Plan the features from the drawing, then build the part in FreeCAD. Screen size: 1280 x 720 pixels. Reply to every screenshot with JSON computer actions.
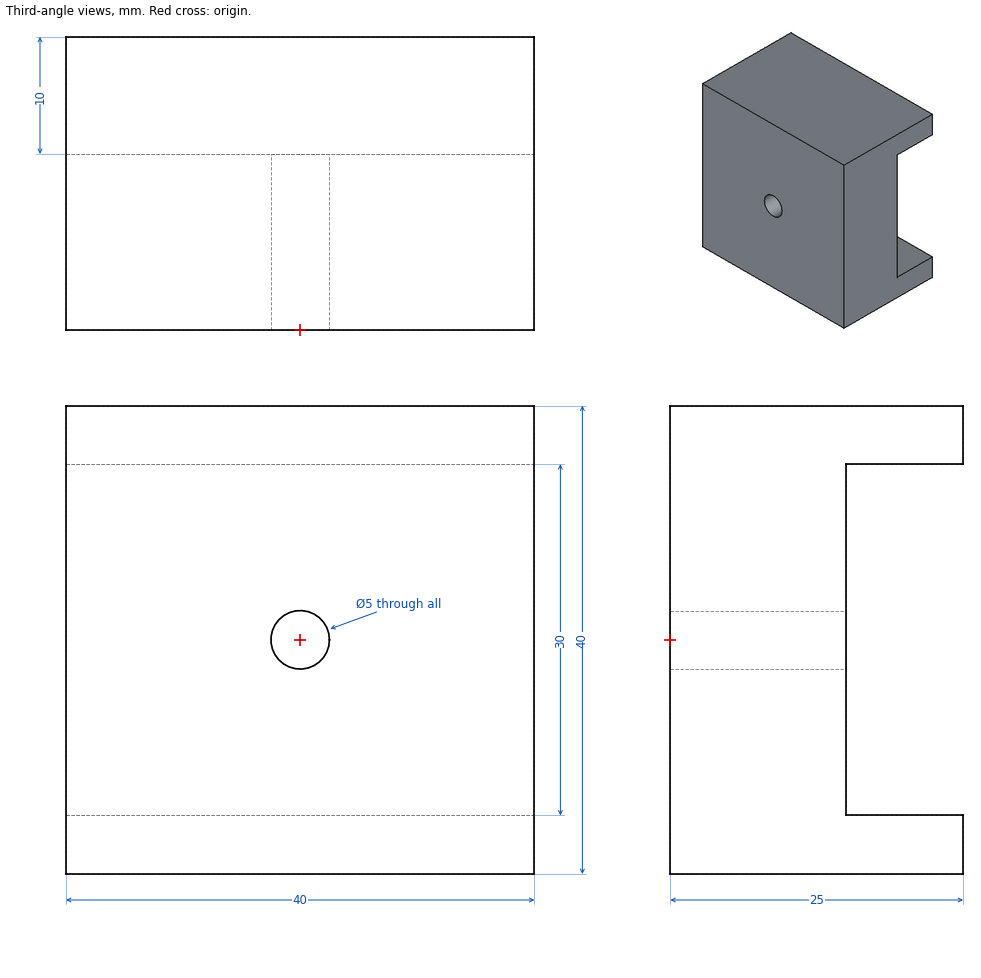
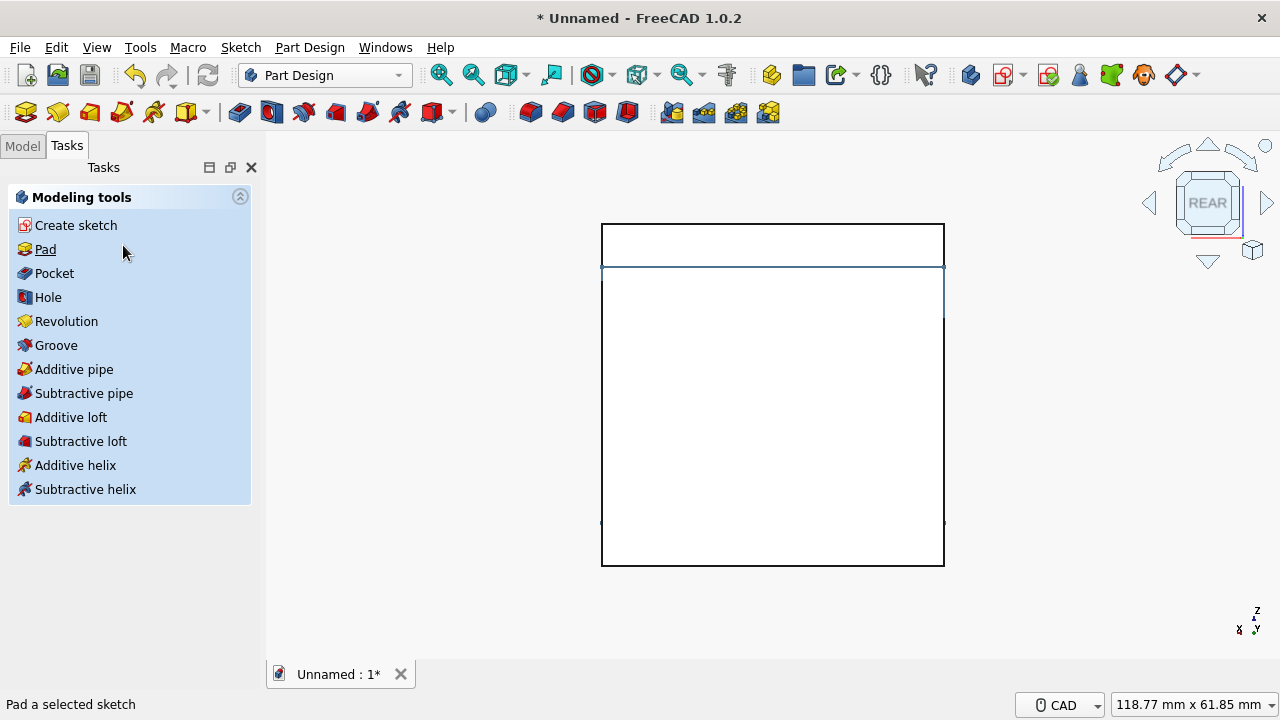
{"action": "left_click", "coordinate": [240, 112]}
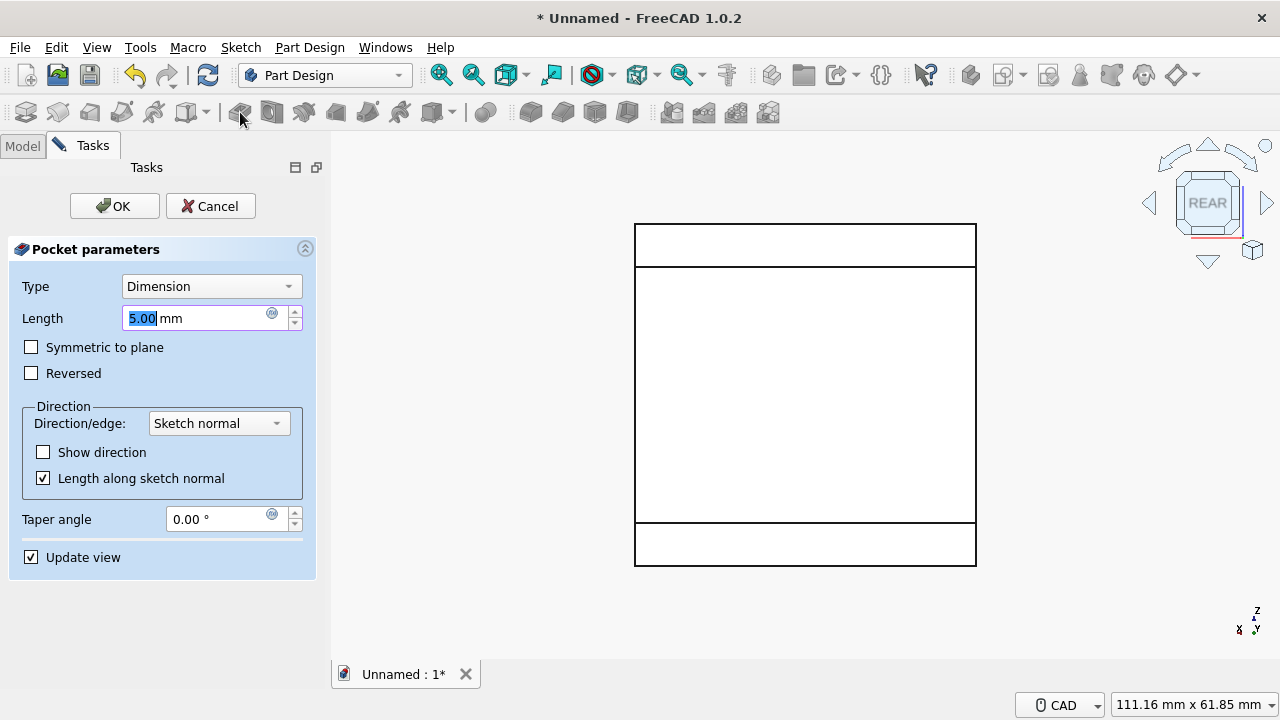
{"action": "type", "text": "10"}
{"action": "key", "text": "Tab"}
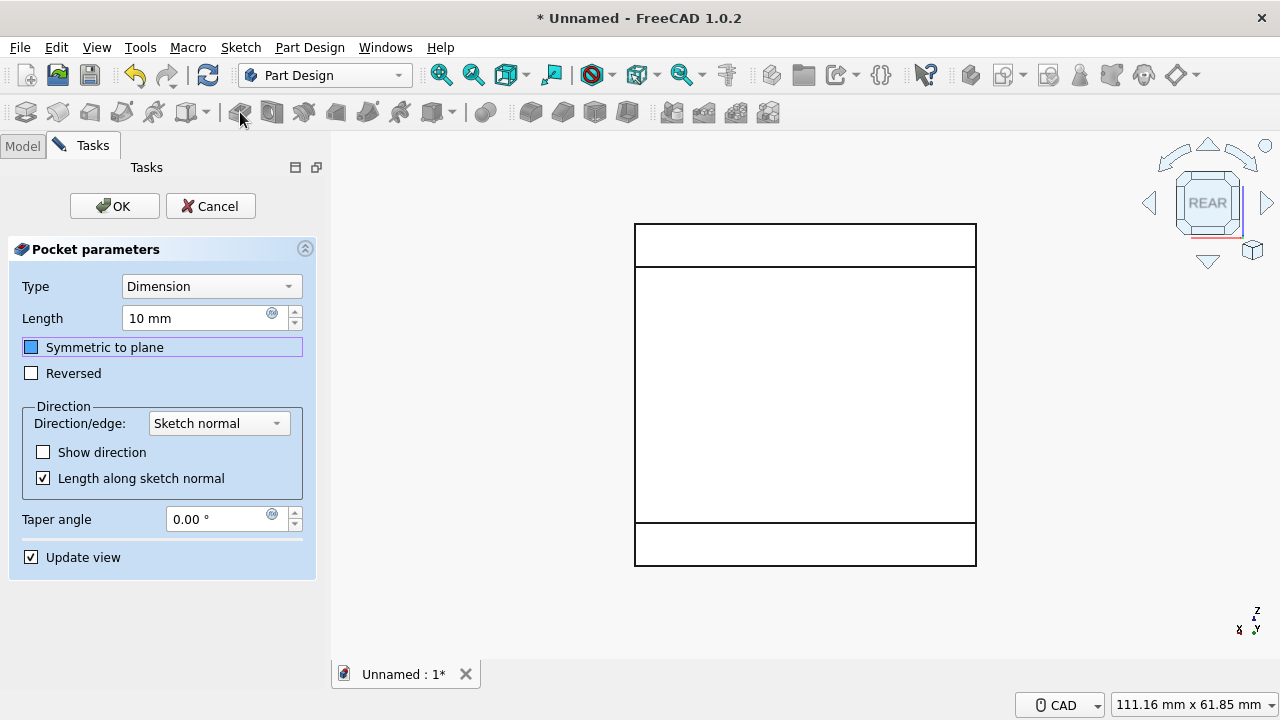
{"action": "left_click", "coordinate": [115, 206]}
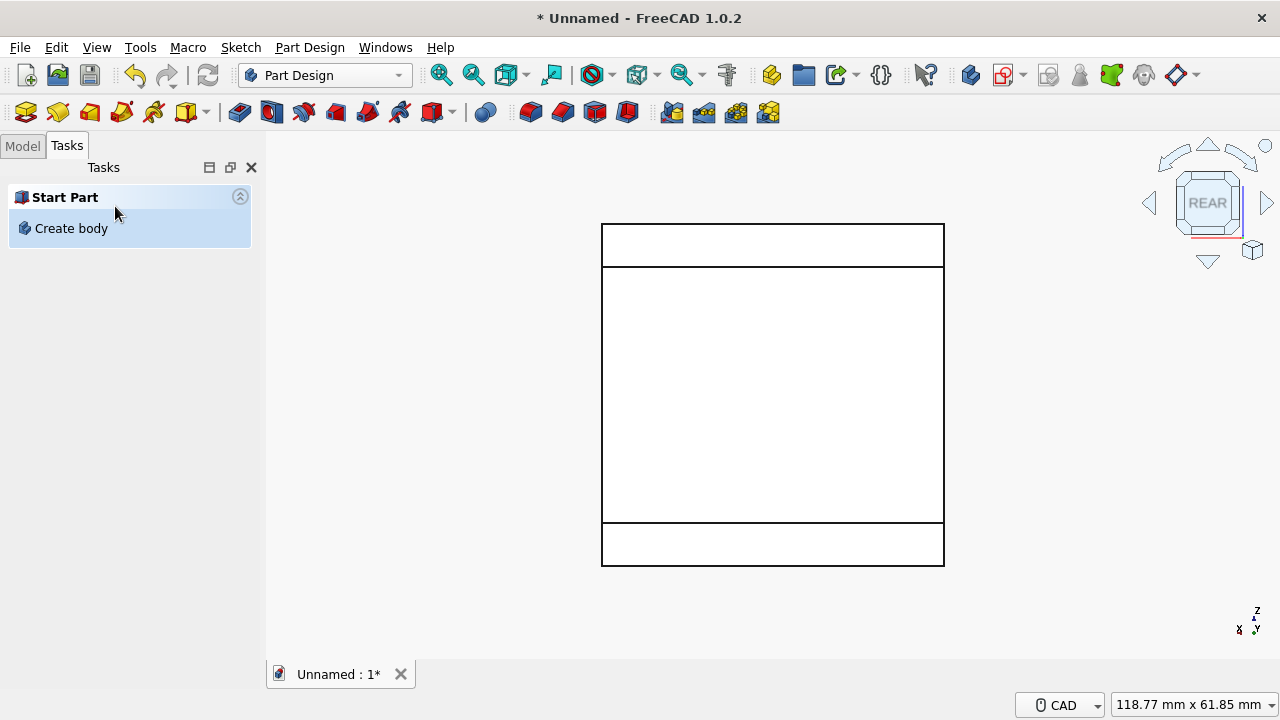
{"action": "left_click", "coordinate": [1004, 76]}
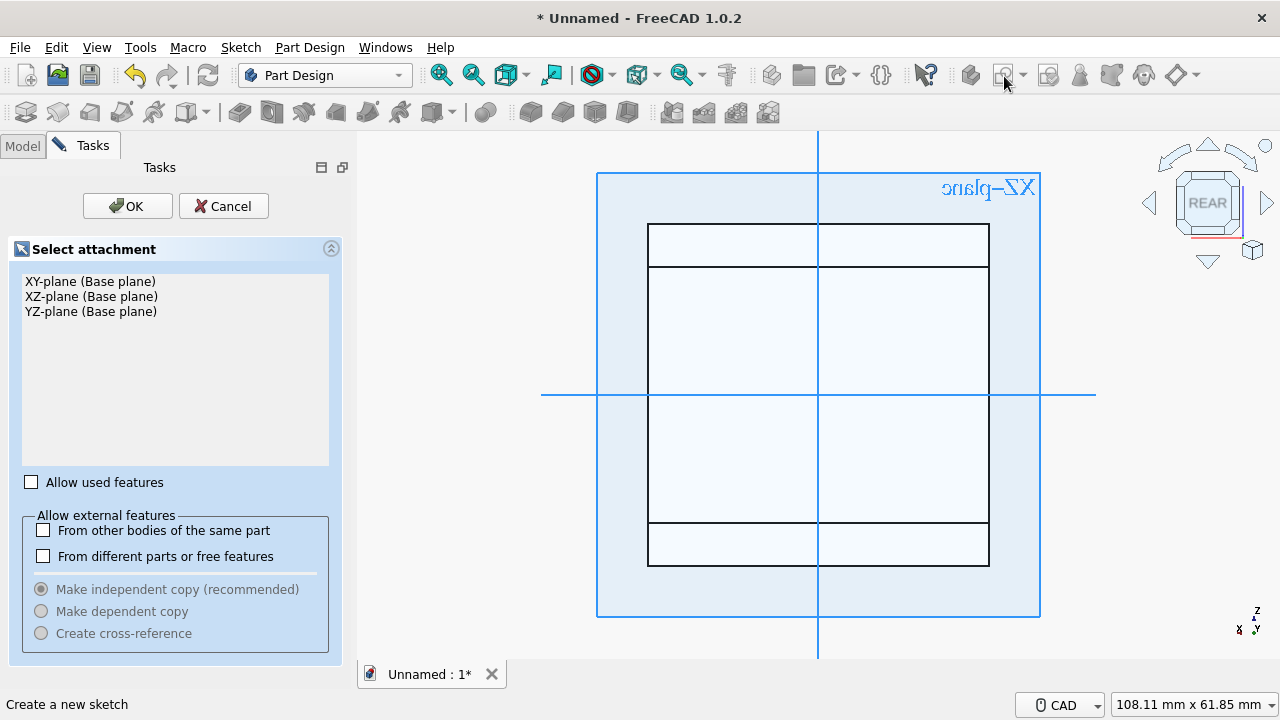
{"action": "left_click", "coordinate": [82, 296]}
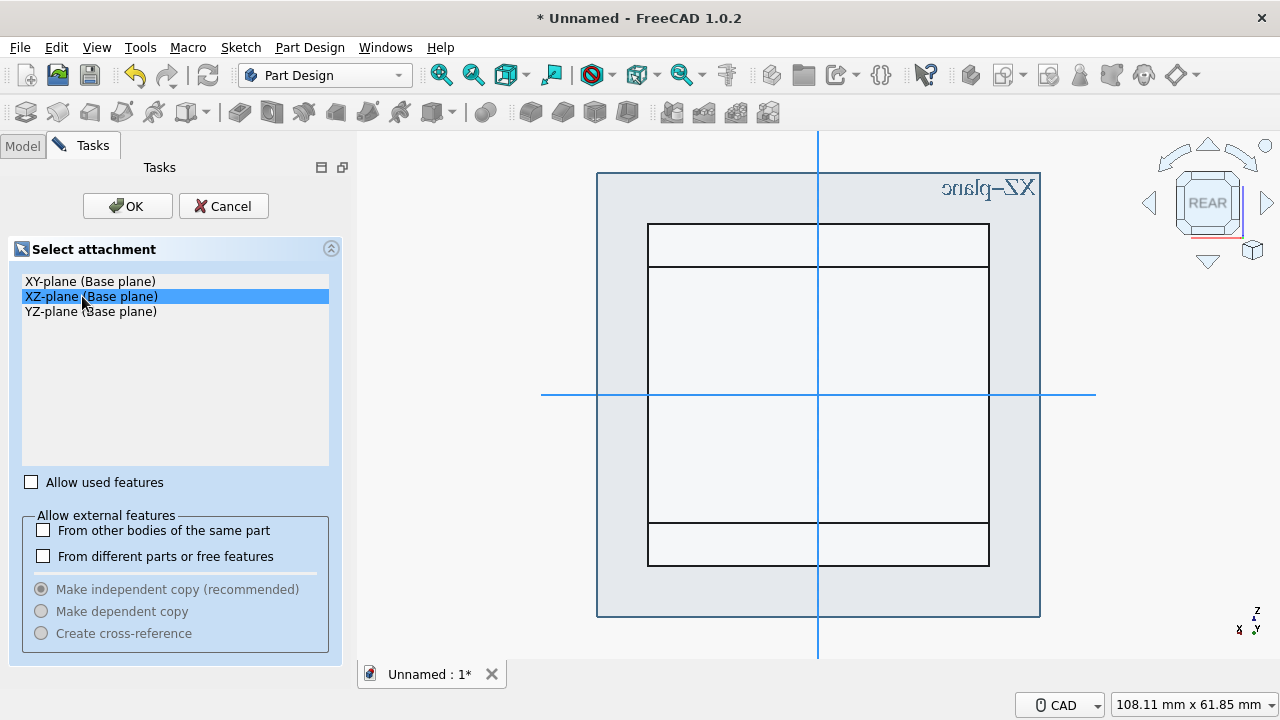
{"action": "left_click", "coordinate": [128, 206]}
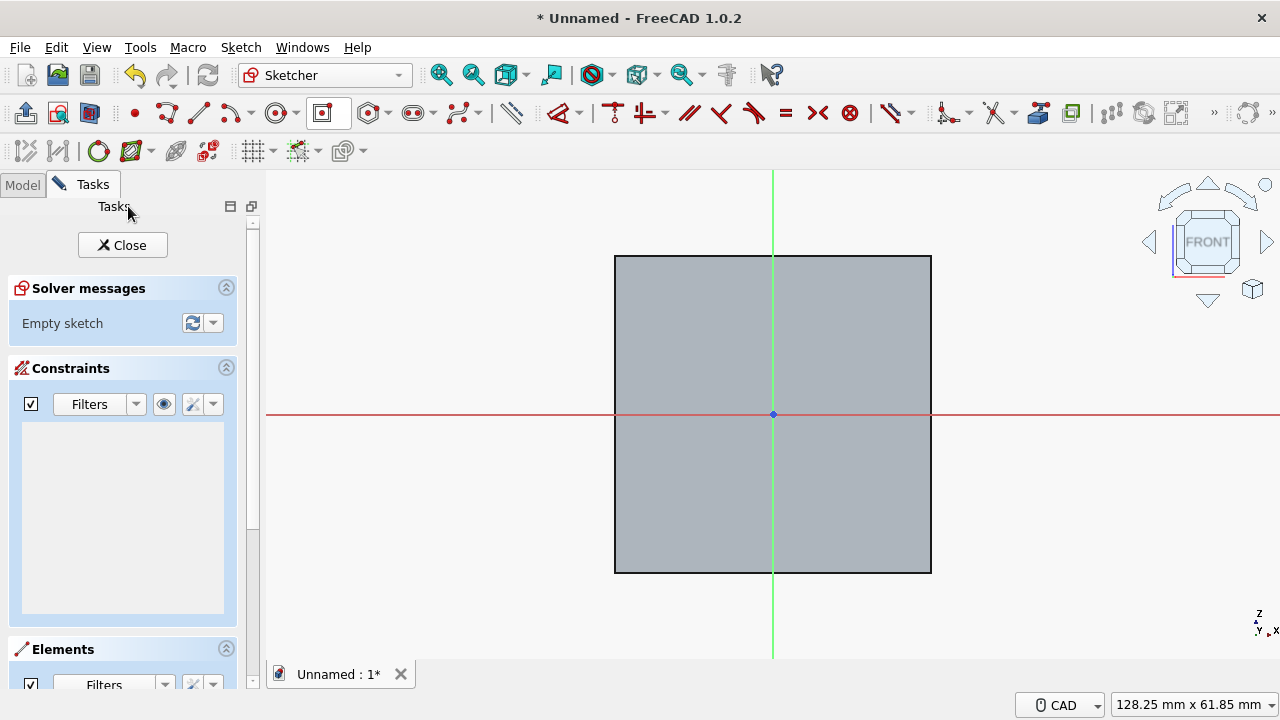
{"action": "scroll", "coordinate": [784, 415], "scroll_direction": "up", "scroll_amount": 10}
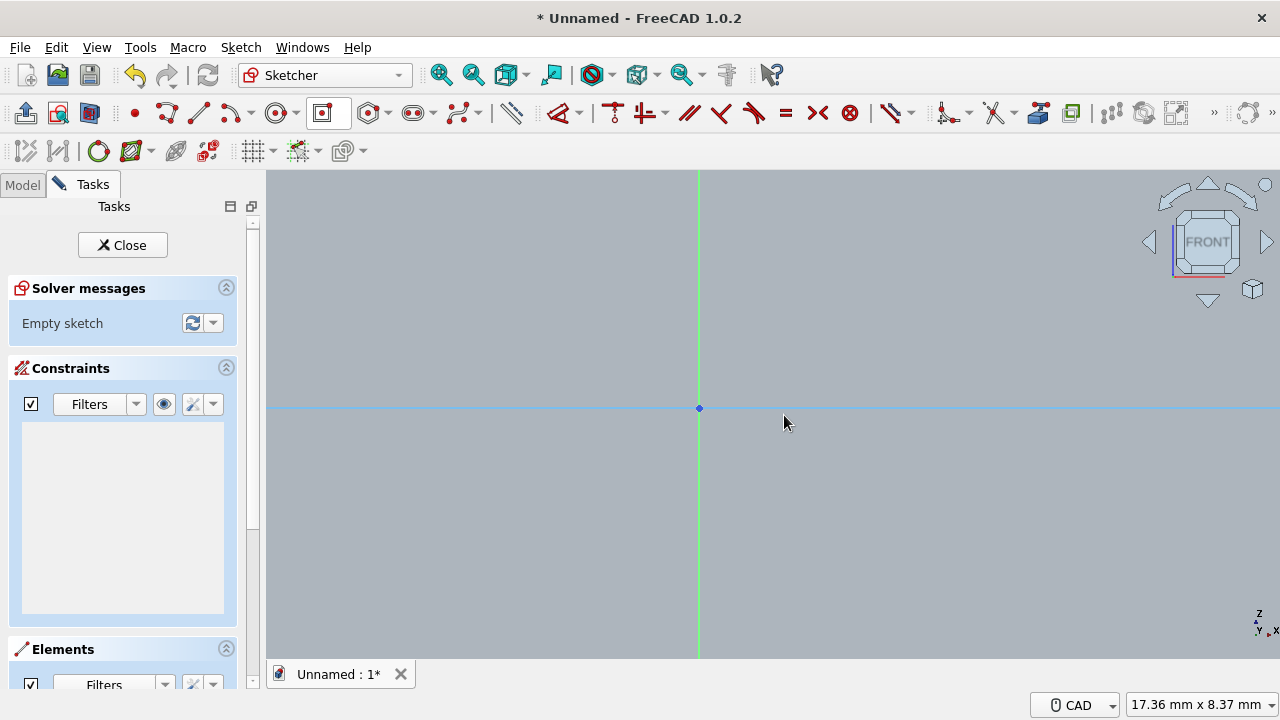
{"action": "left_click", "coordinate": [276, 114]}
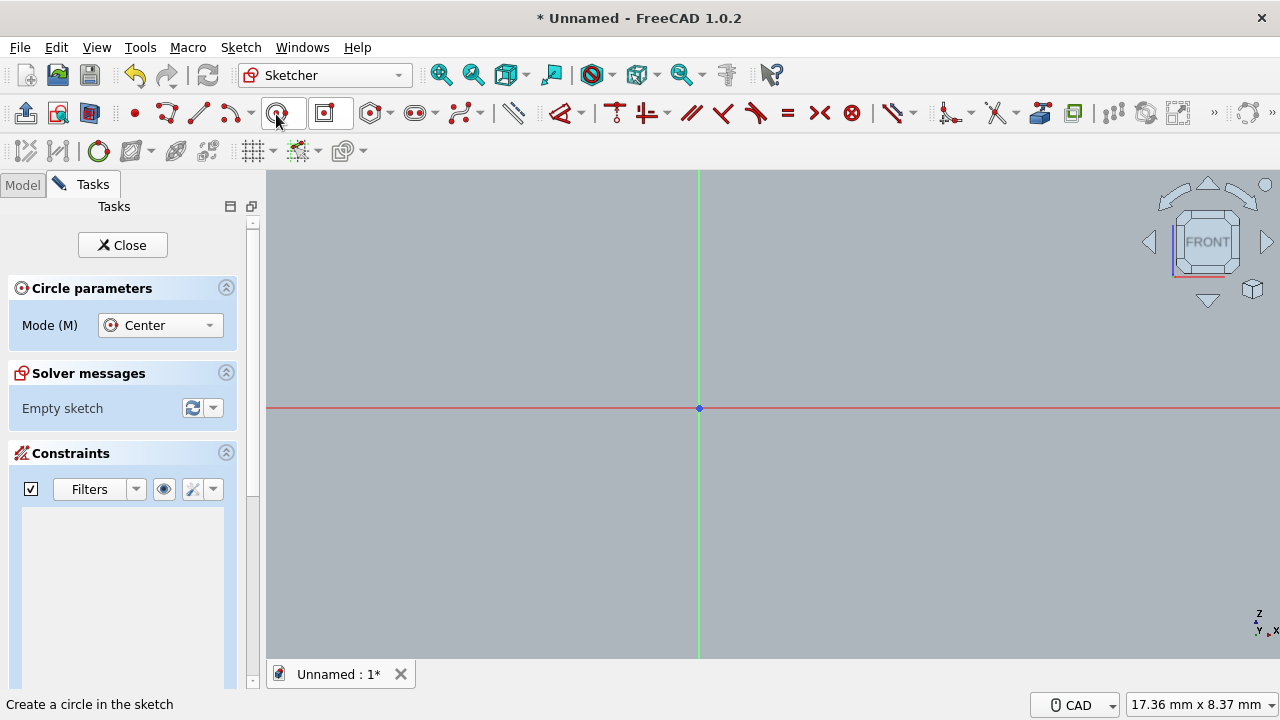
{"action": "left_click", "coordinate": [699, 408]}
{"action": "mouse_move", "coordinate": [803, 305]}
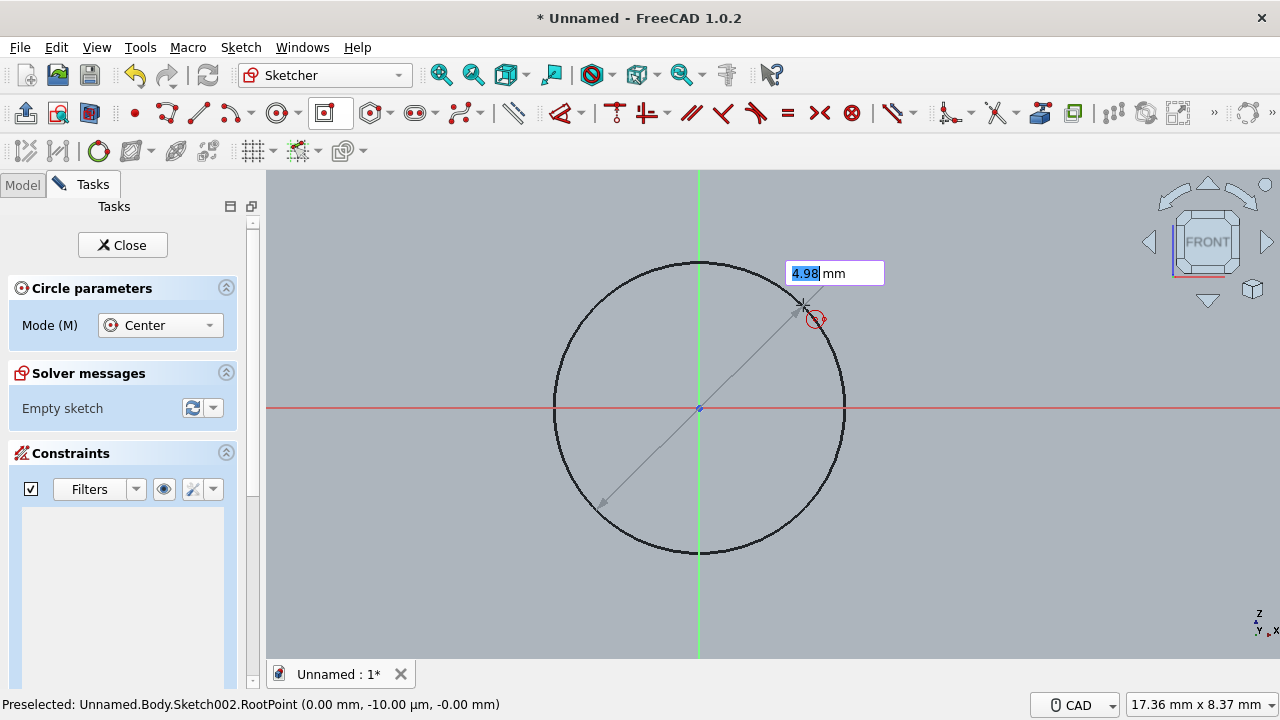
{"action": "type", "text": "5"}
{"action": "key", "text": "Return"}
{"action": "key", "text": "Escape"}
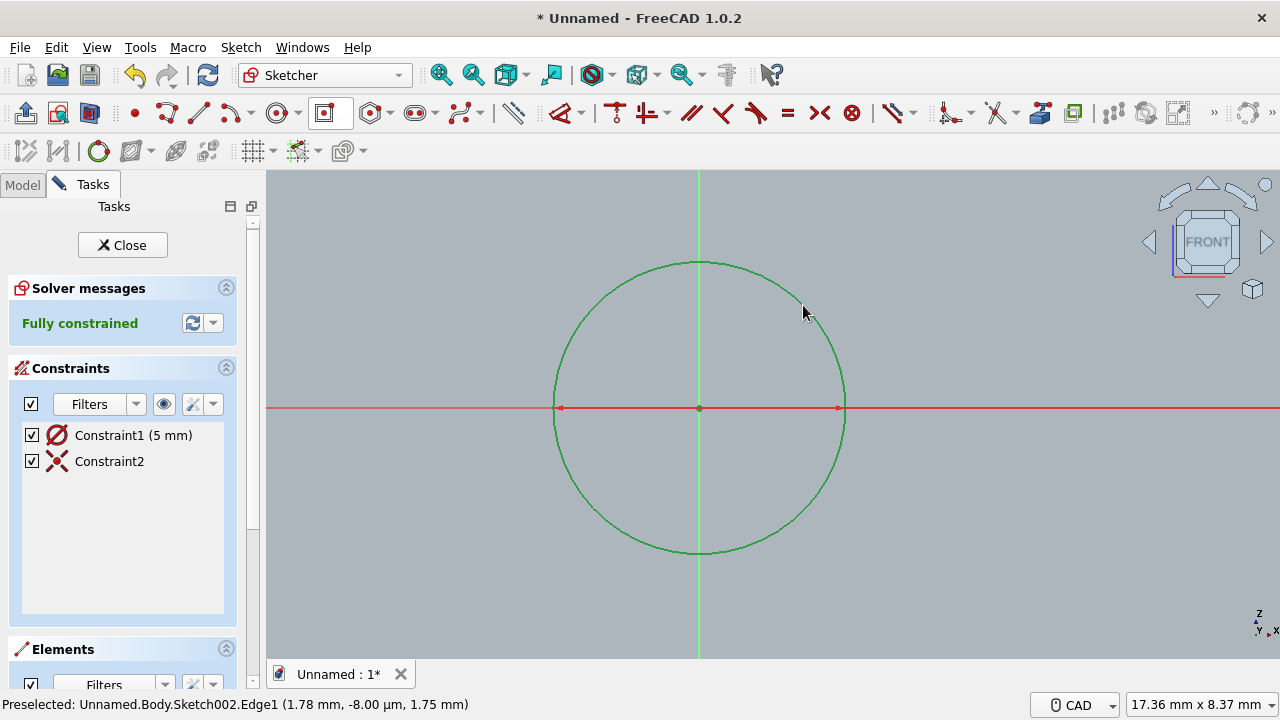
{"action": "left_click", "coordinate": [123, 245]}